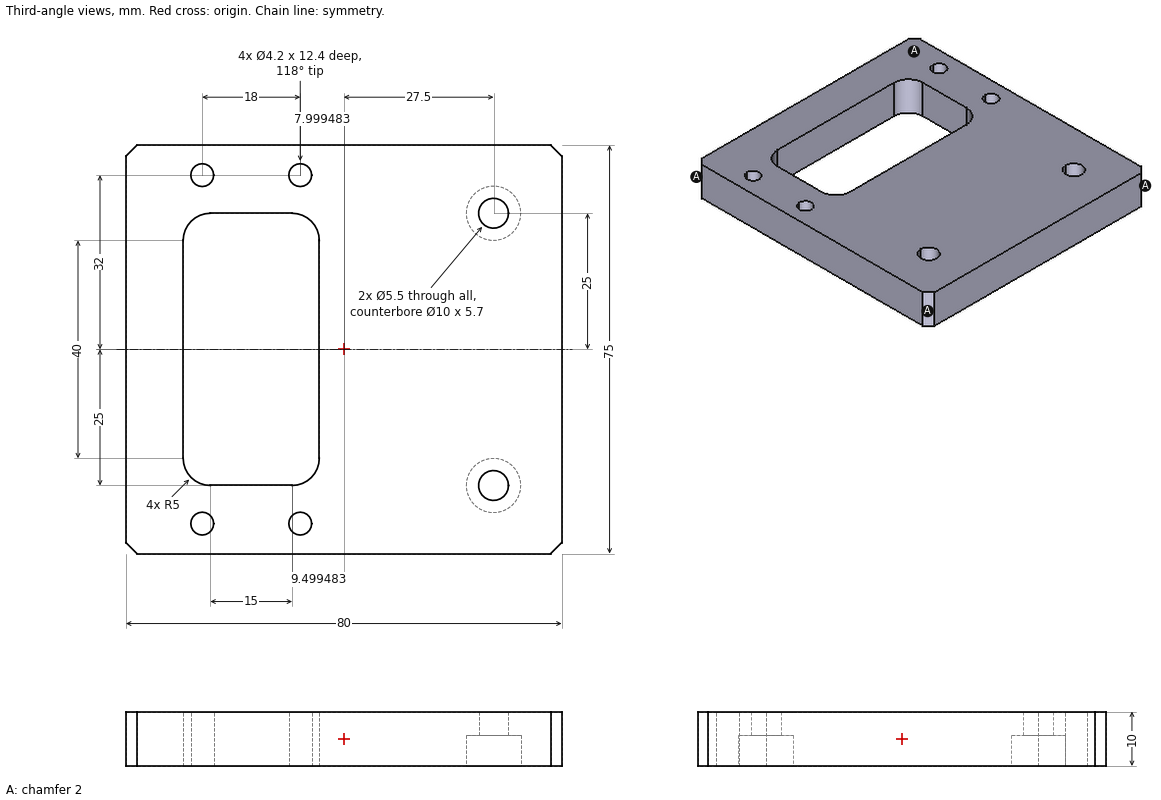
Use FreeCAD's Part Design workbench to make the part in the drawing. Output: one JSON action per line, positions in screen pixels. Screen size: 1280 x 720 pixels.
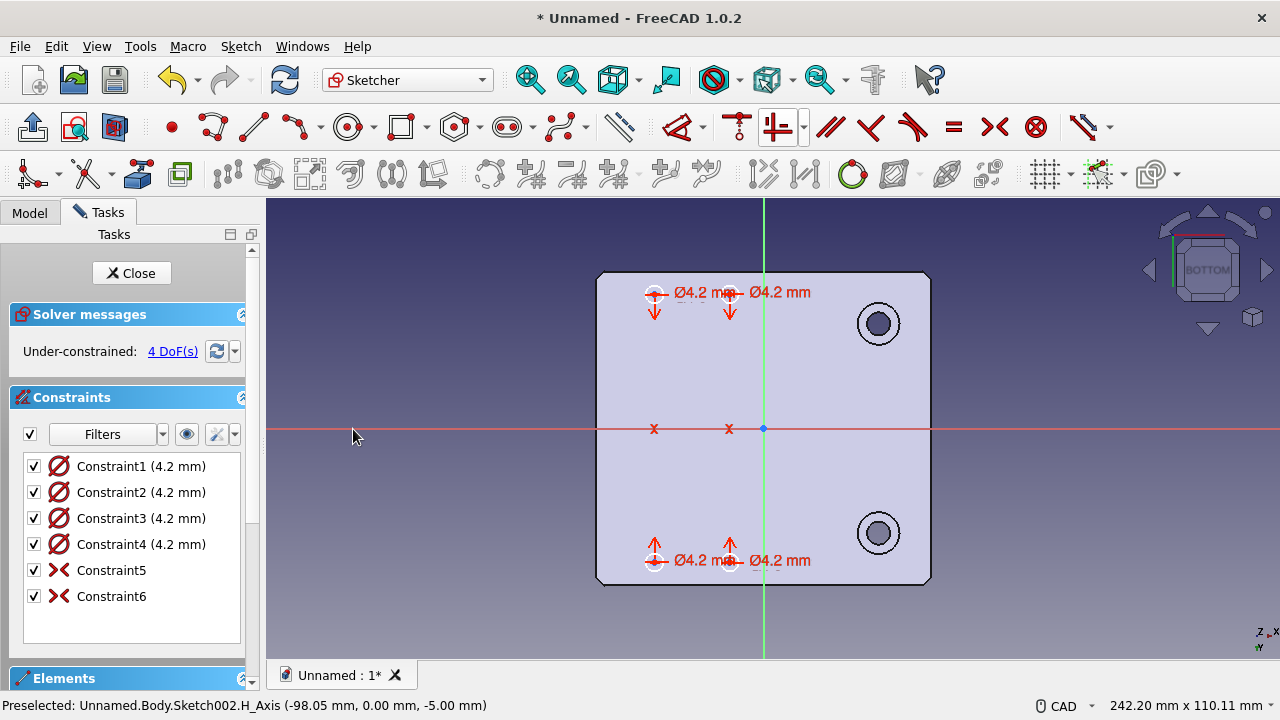
{"action": "left_click", "coordinate": [730, 563]}
{"action": "left_click", "coordinate": [798, 496]}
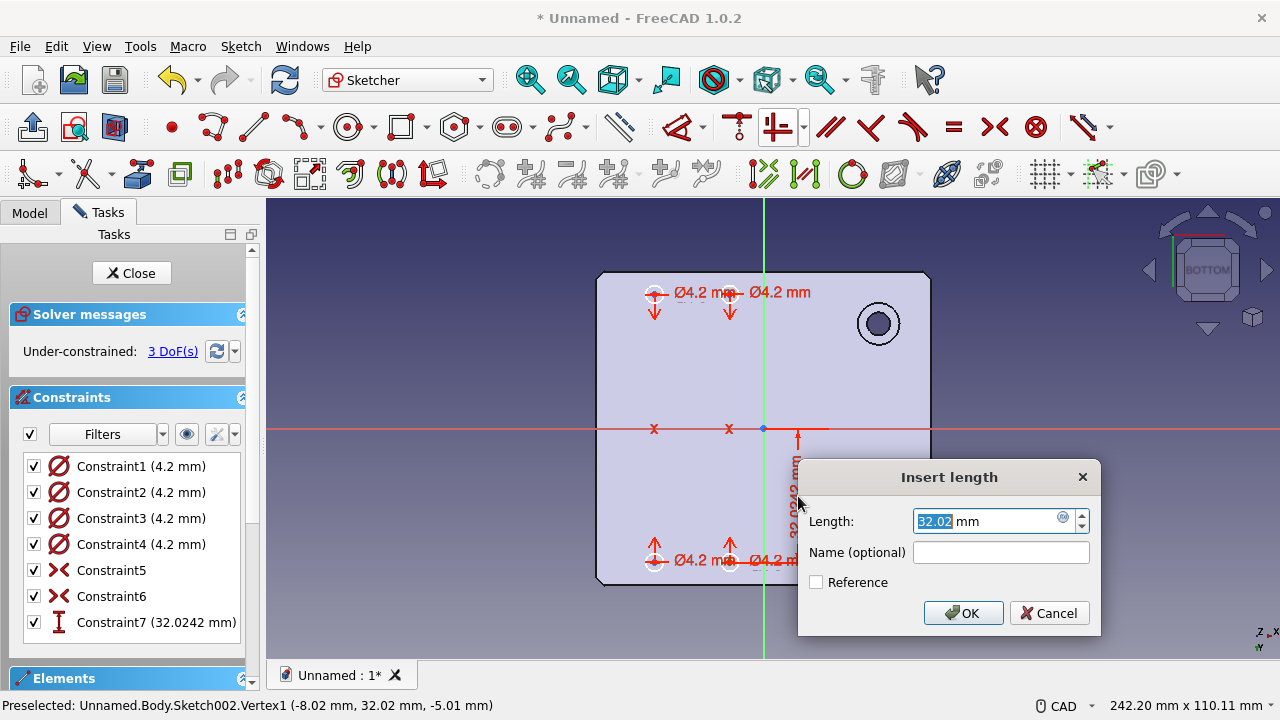
{"action": "type", "text": "32"}
{"action": "key", "text": "Return"}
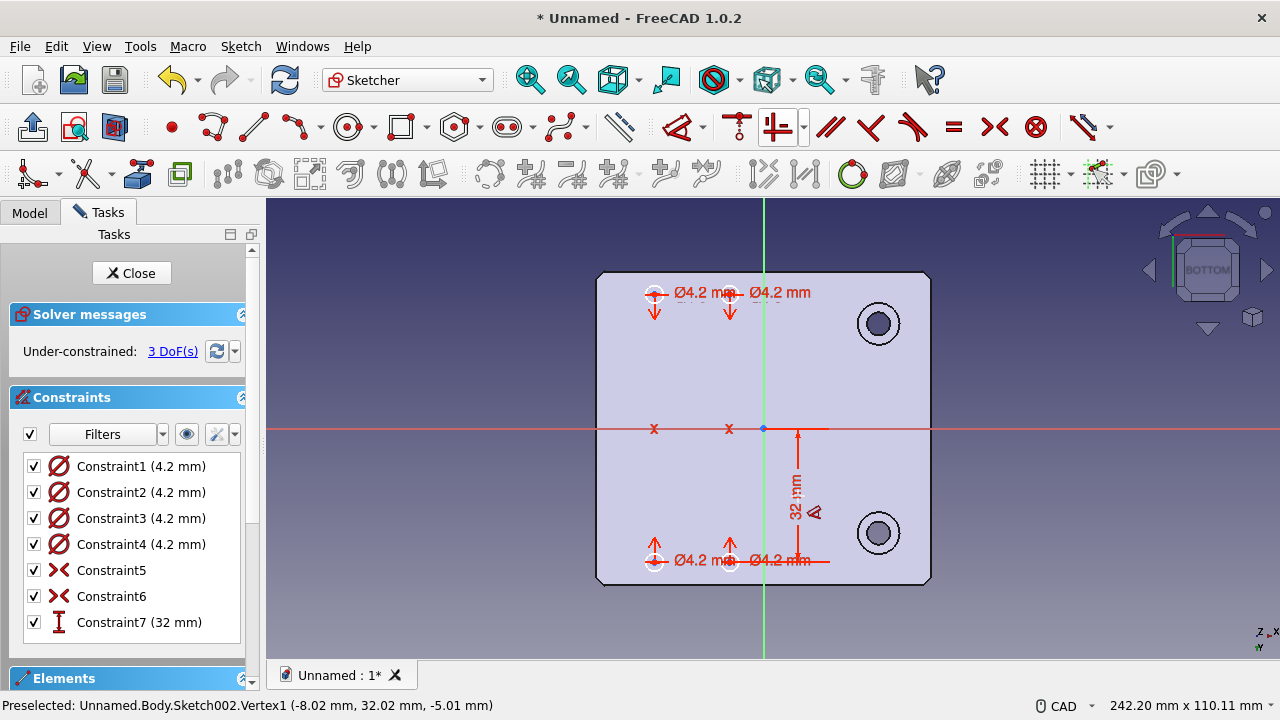
{"action": "left_click", "coordinate": [655, 562]}
{"action": "left_click", "coordinate": [798, 465]}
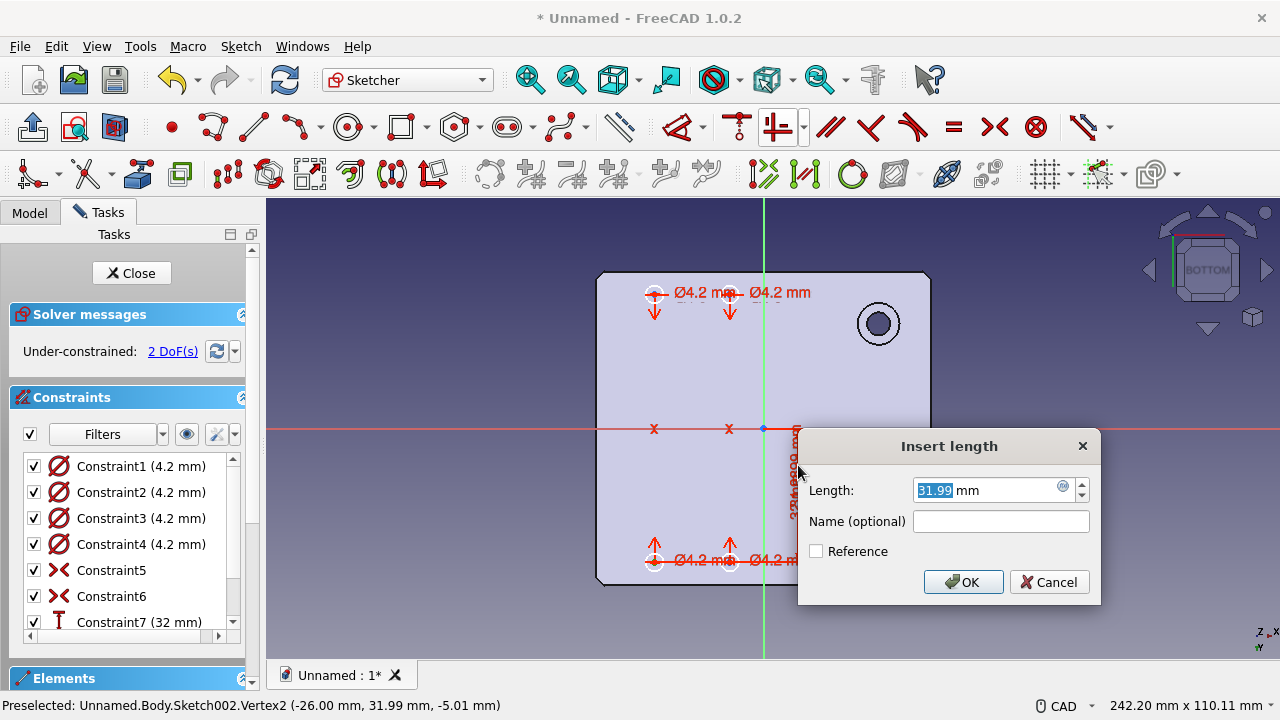
{"action": "type", "text": "32"}
{"action": "key", "text": "Return"}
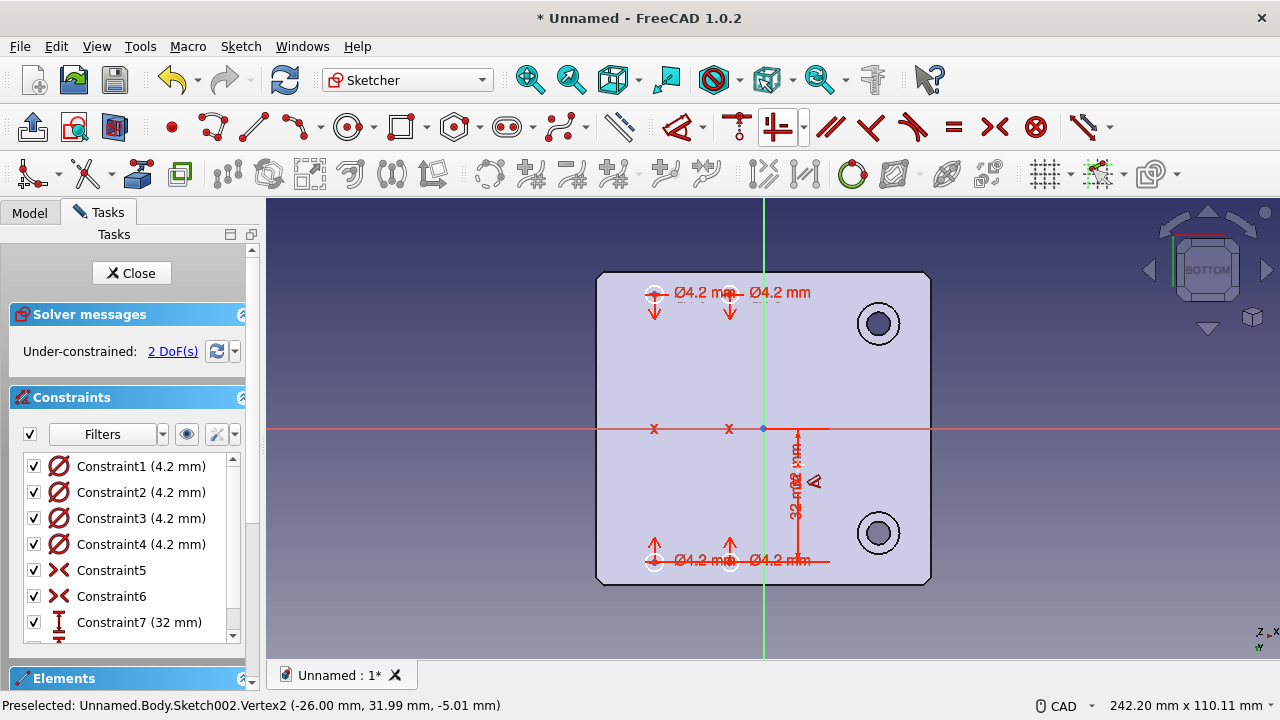
{"action": "left_click", "coordinate": [730, 562]}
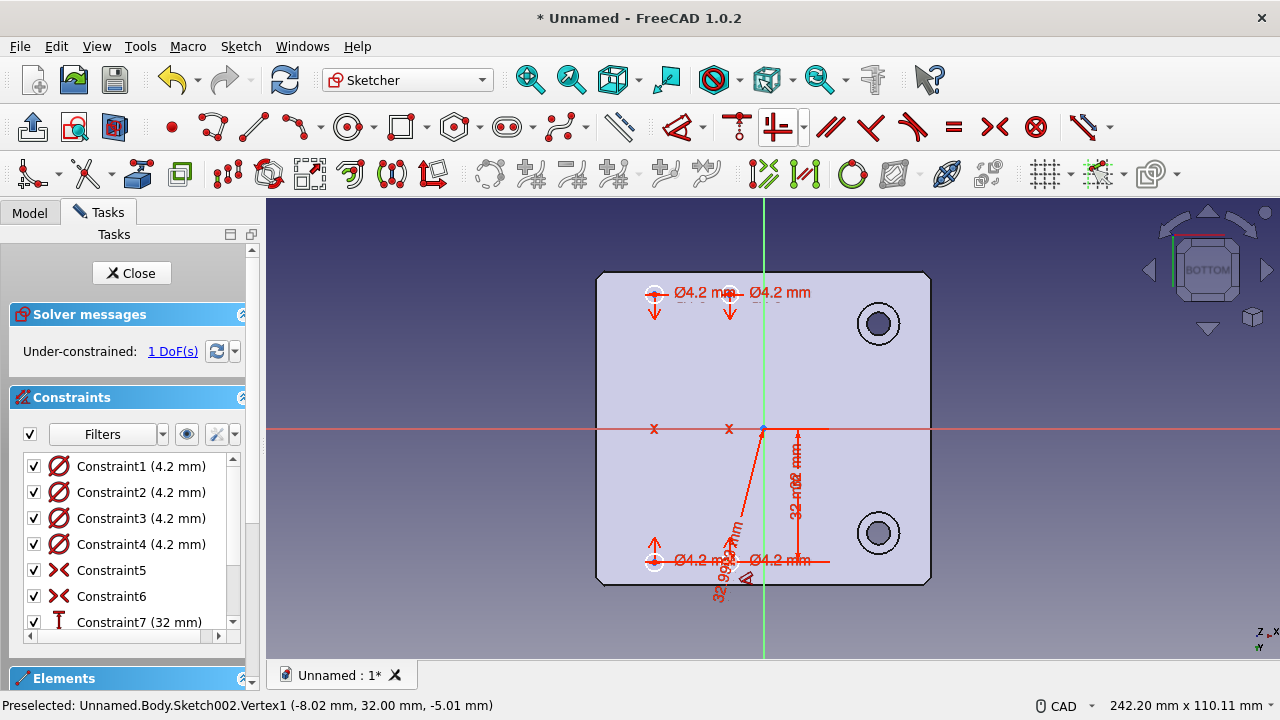
{"action": "left_click", "coordinate": [655, 562]}
{"action": "left_click", "coordinate": [692, 596]}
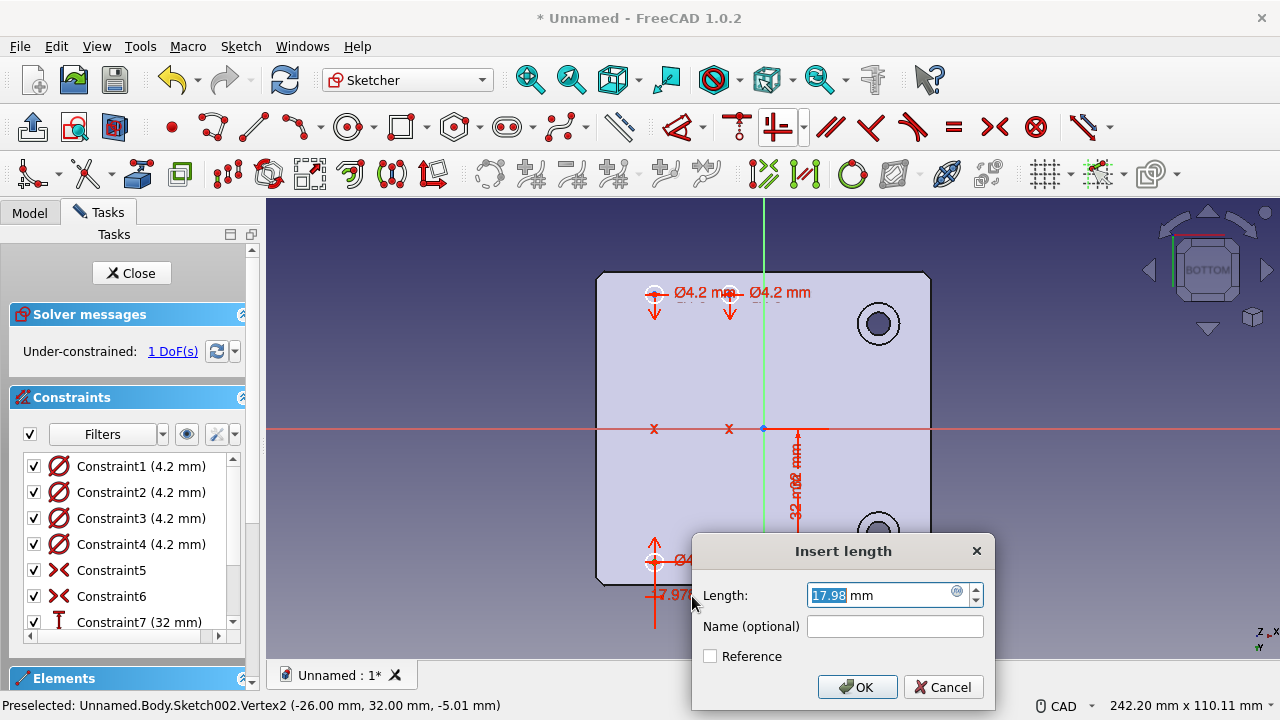
{"action": "type", "text": "18"}
{"action": "key", "text": "Return"}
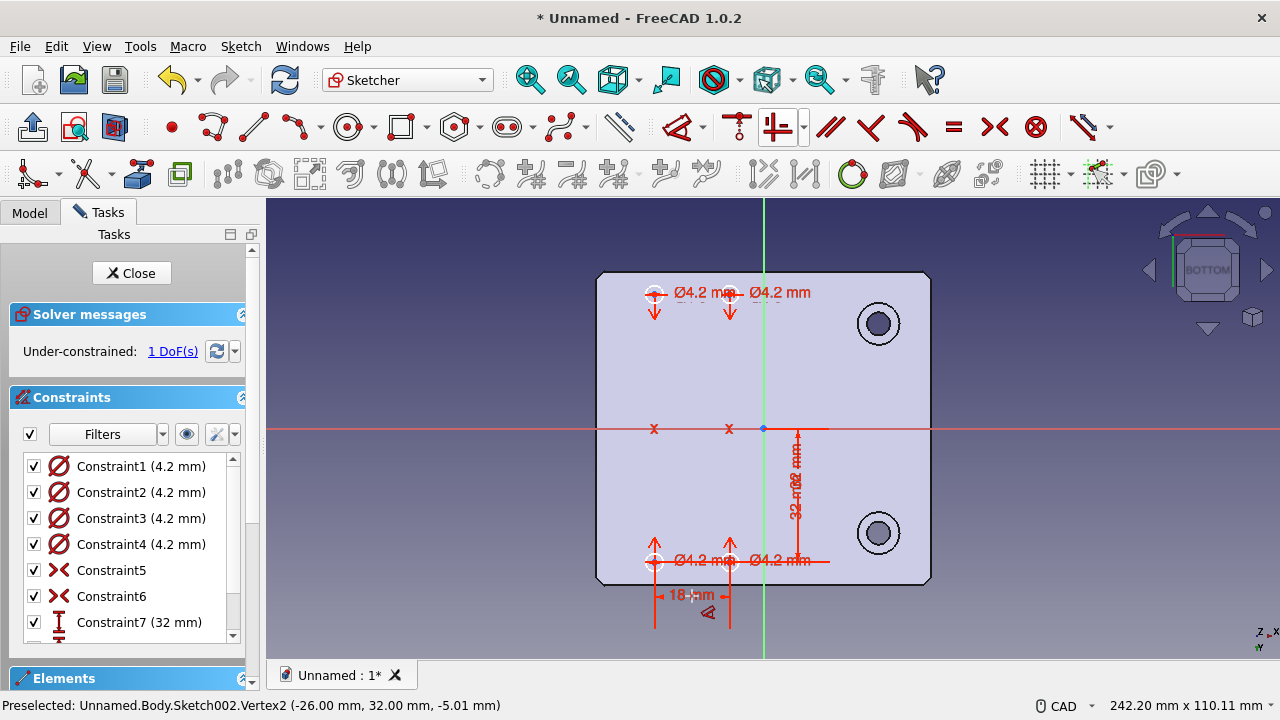
{"action": "left_click", "coordinate": [730, 562]}
{"action": "left_click", "coordinate": [747, 395]}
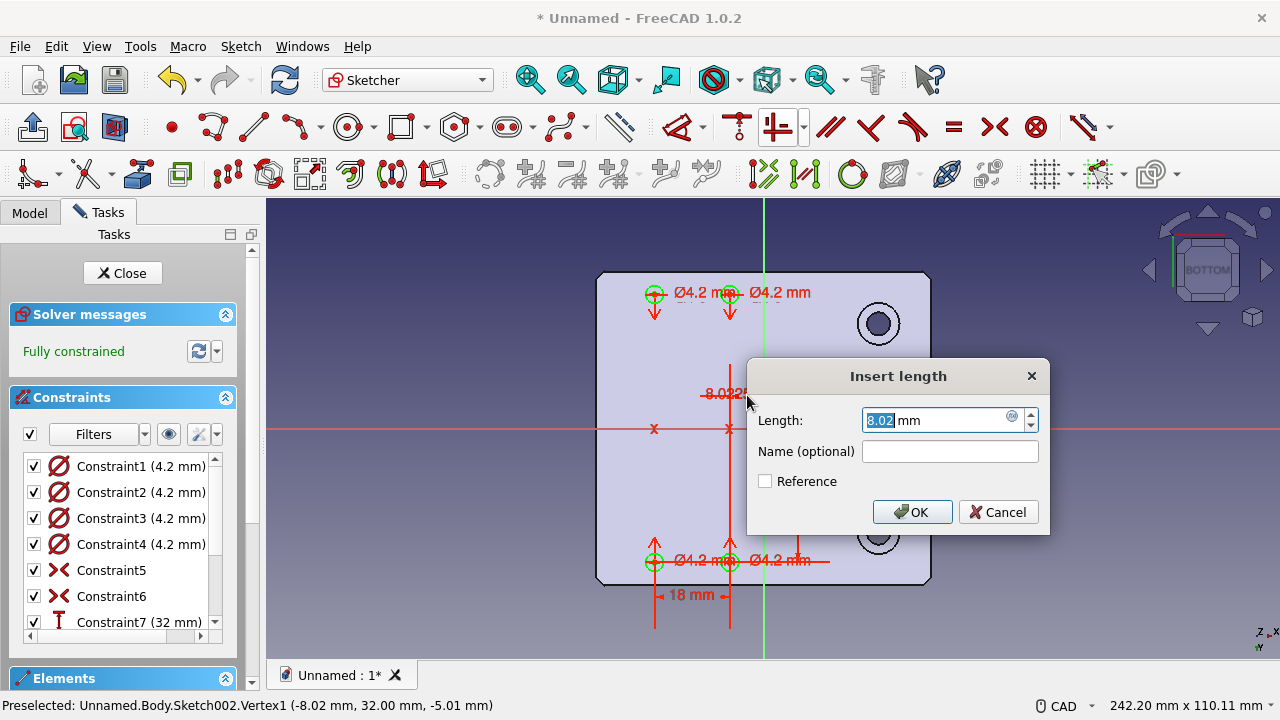
{"action": "type", "text": "7.999483"}
{"action": "key", "text": "Return"}
{"action": "key", "text": "Escape"}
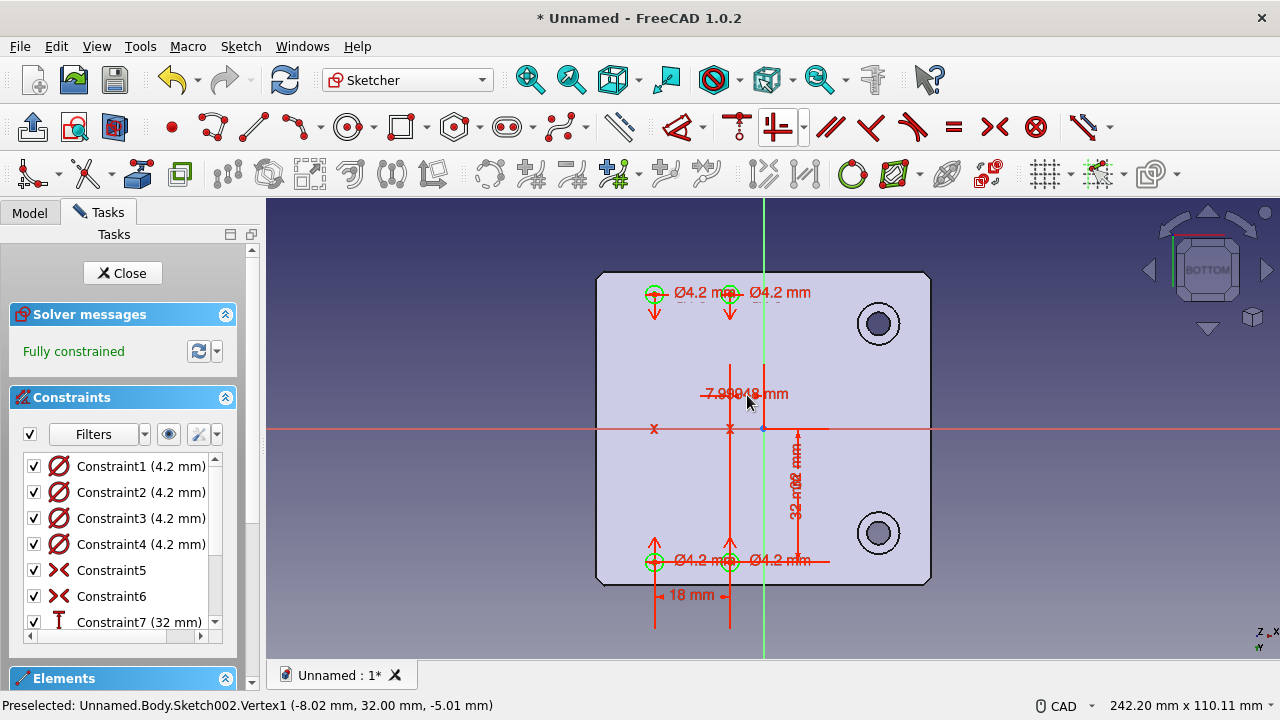
{"action": "left_click", "coordinate": [123, 273]}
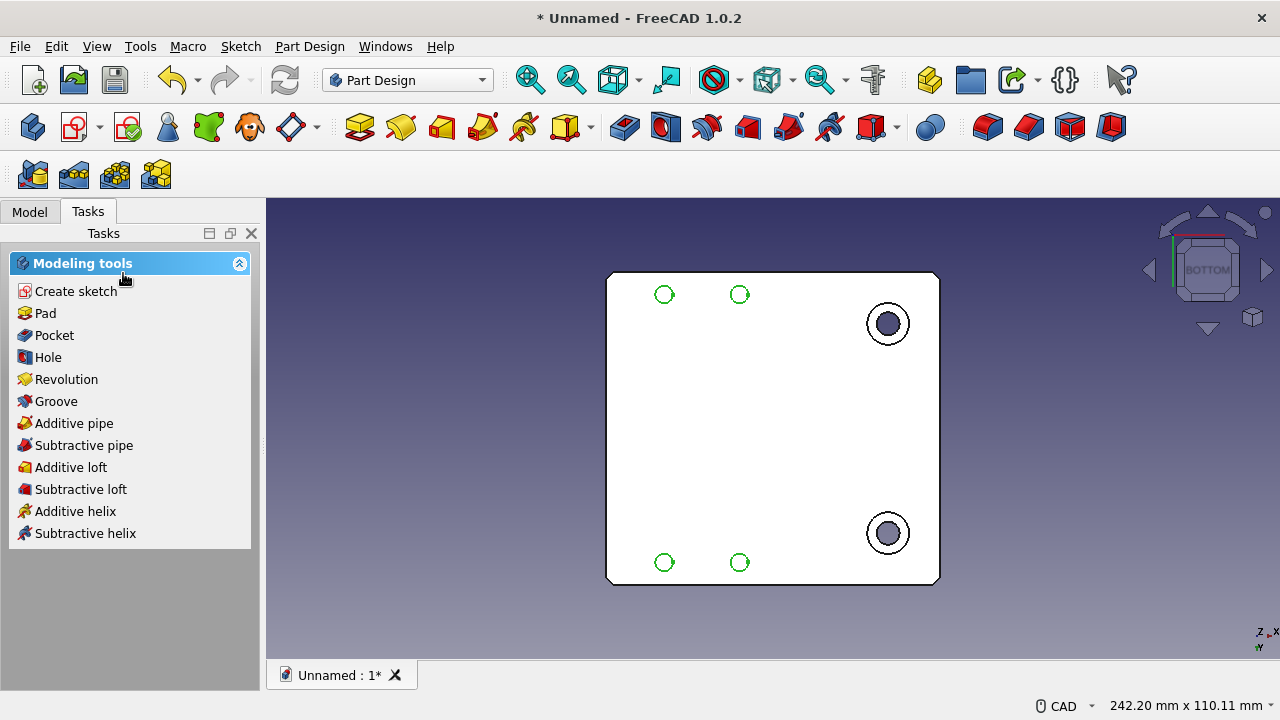
{"action": "left_click", "coordinate": [666, 128]}